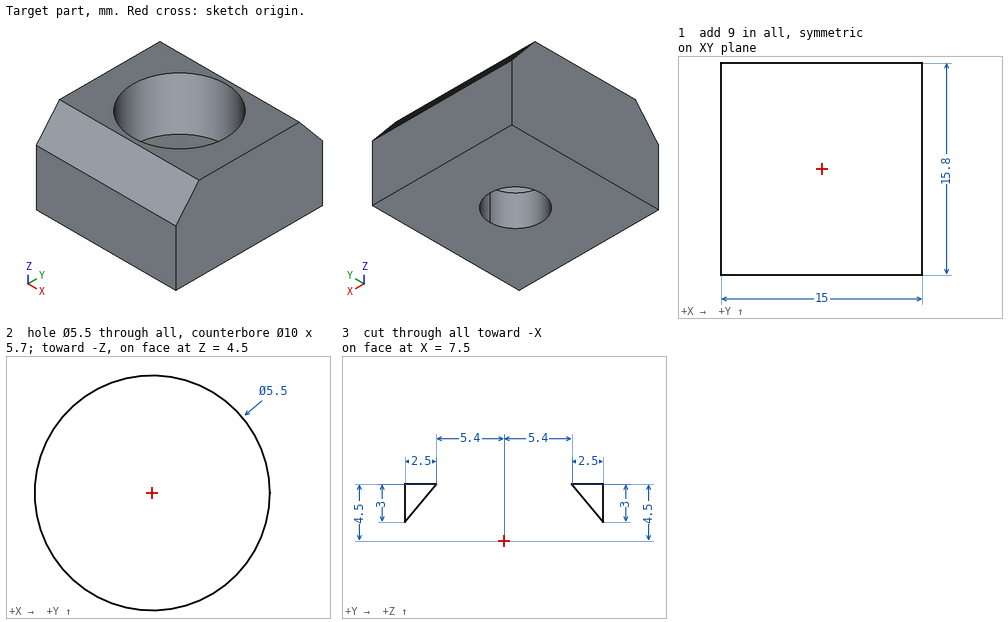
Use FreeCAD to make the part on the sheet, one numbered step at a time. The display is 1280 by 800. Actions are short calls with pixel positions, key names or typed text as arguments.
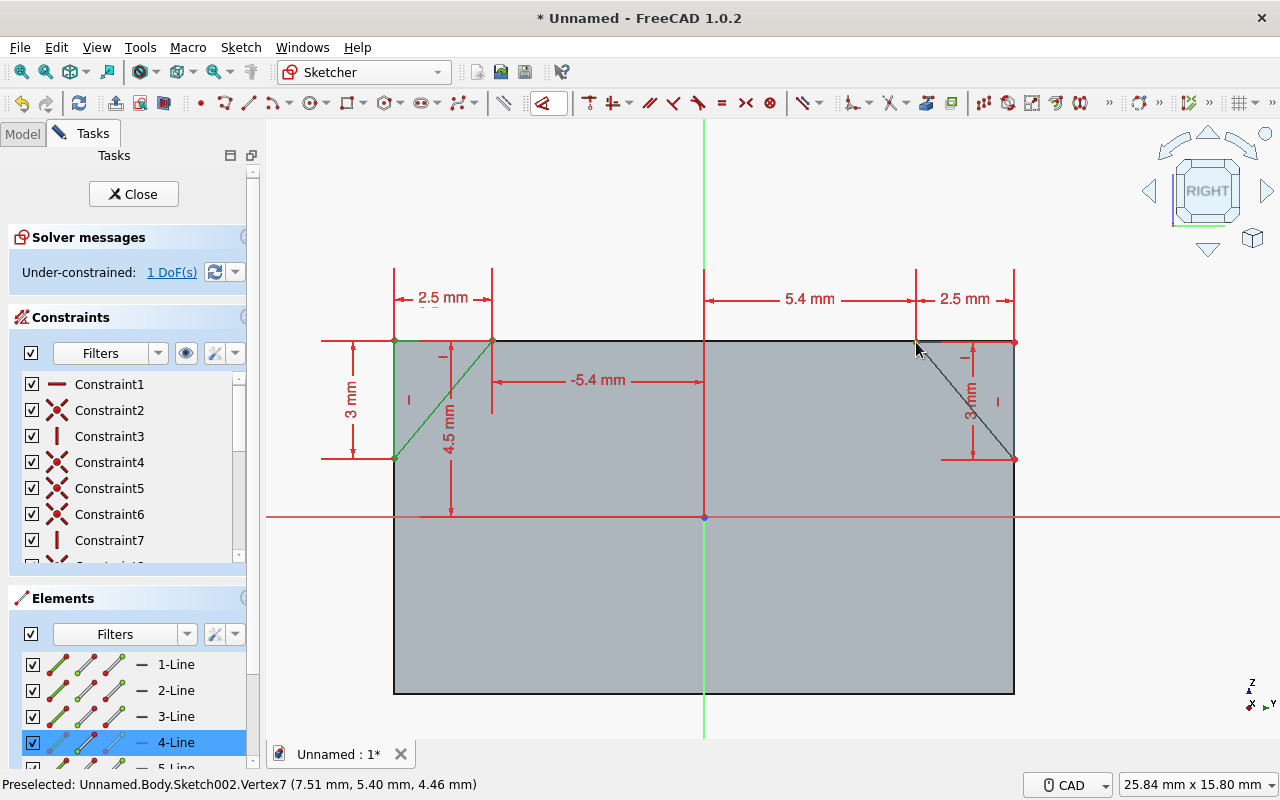
key(i)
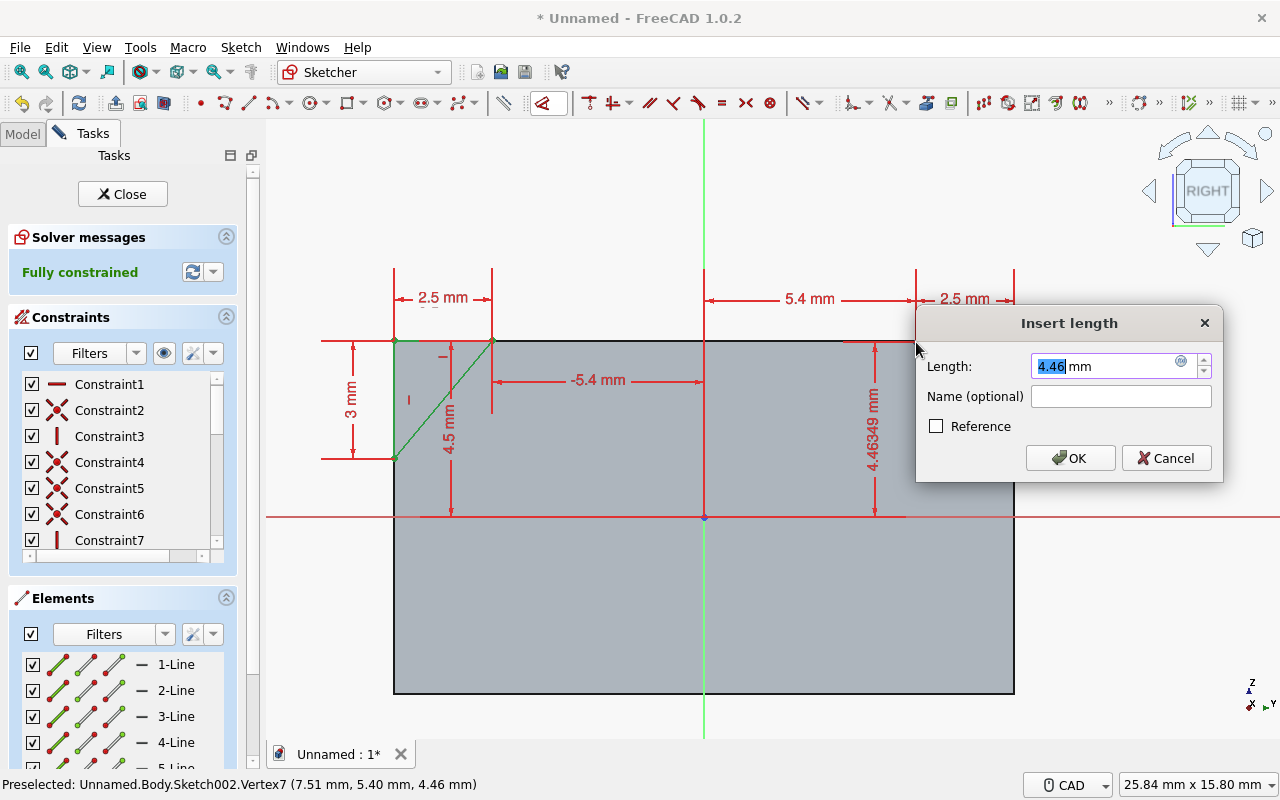
text(4.5)
key(Return)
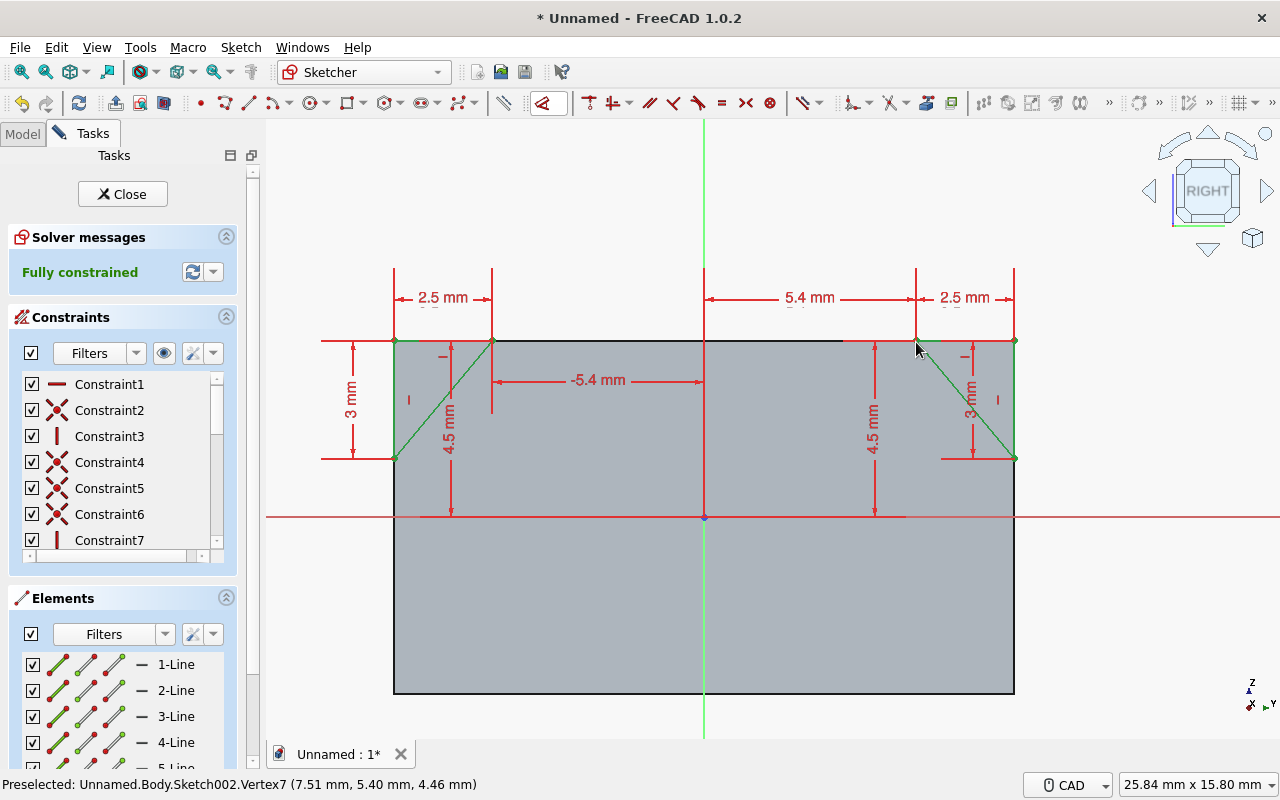
click(123, 194)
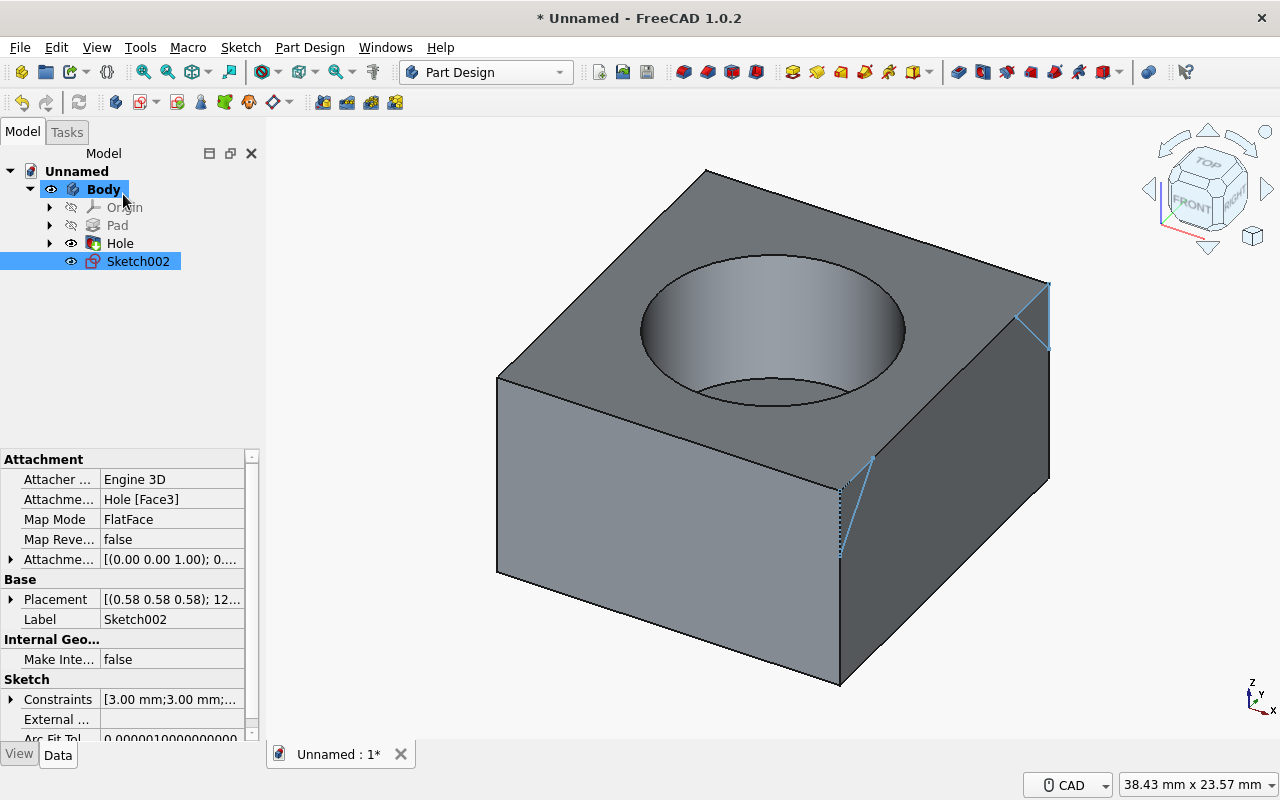
click(960, 72)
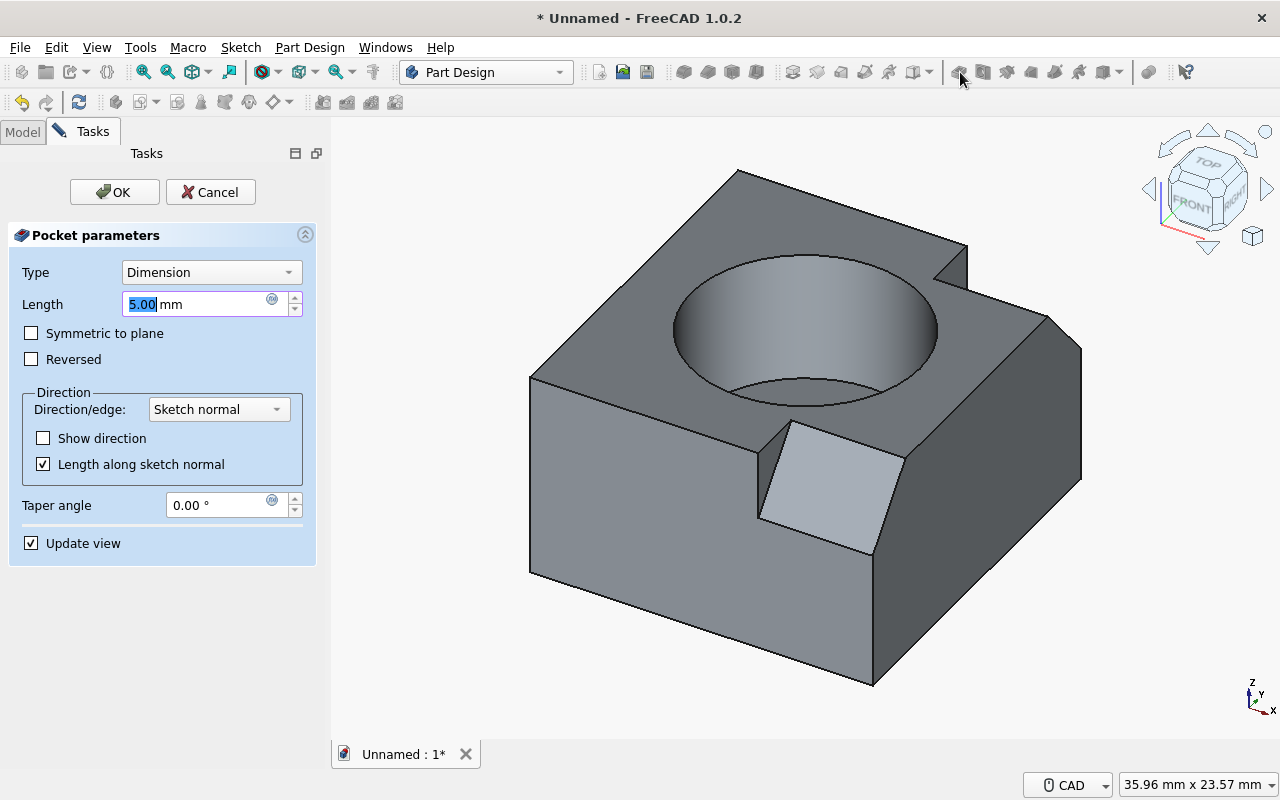
click(212, 272)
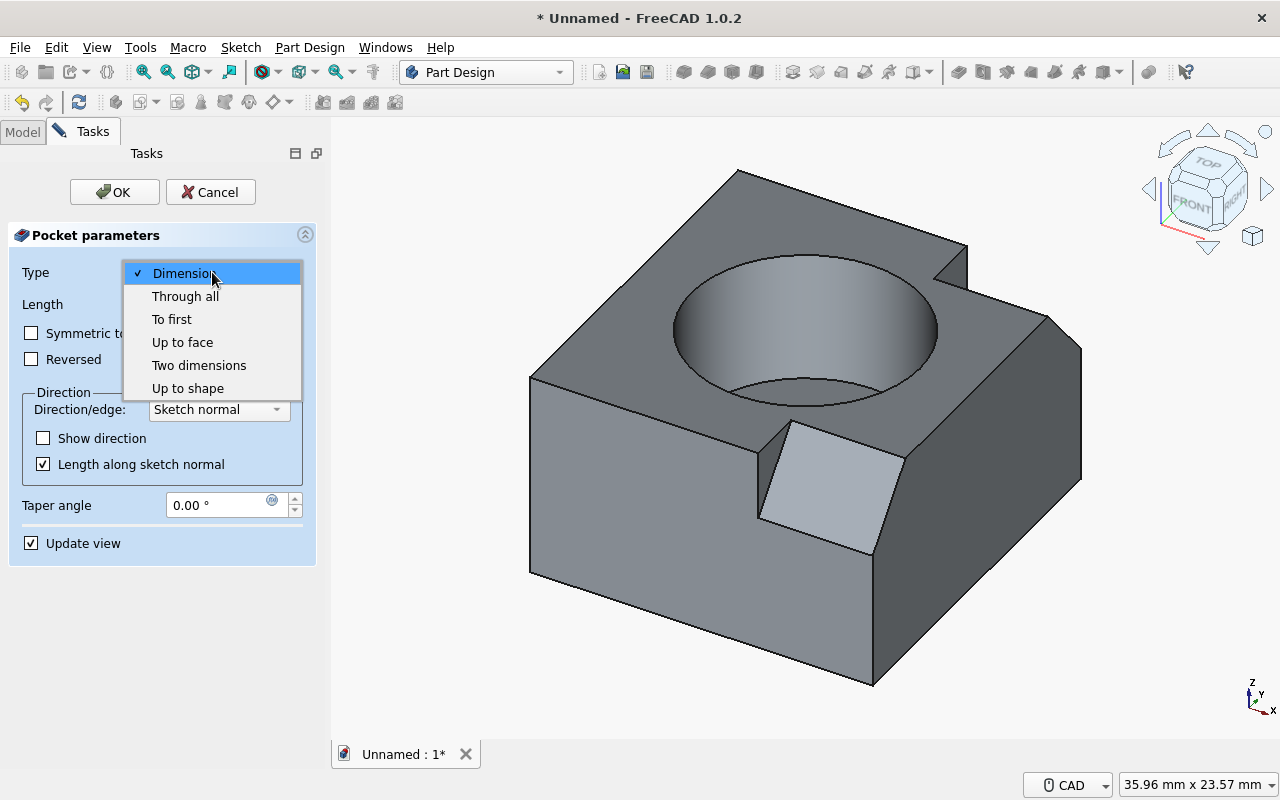
click(212, 296)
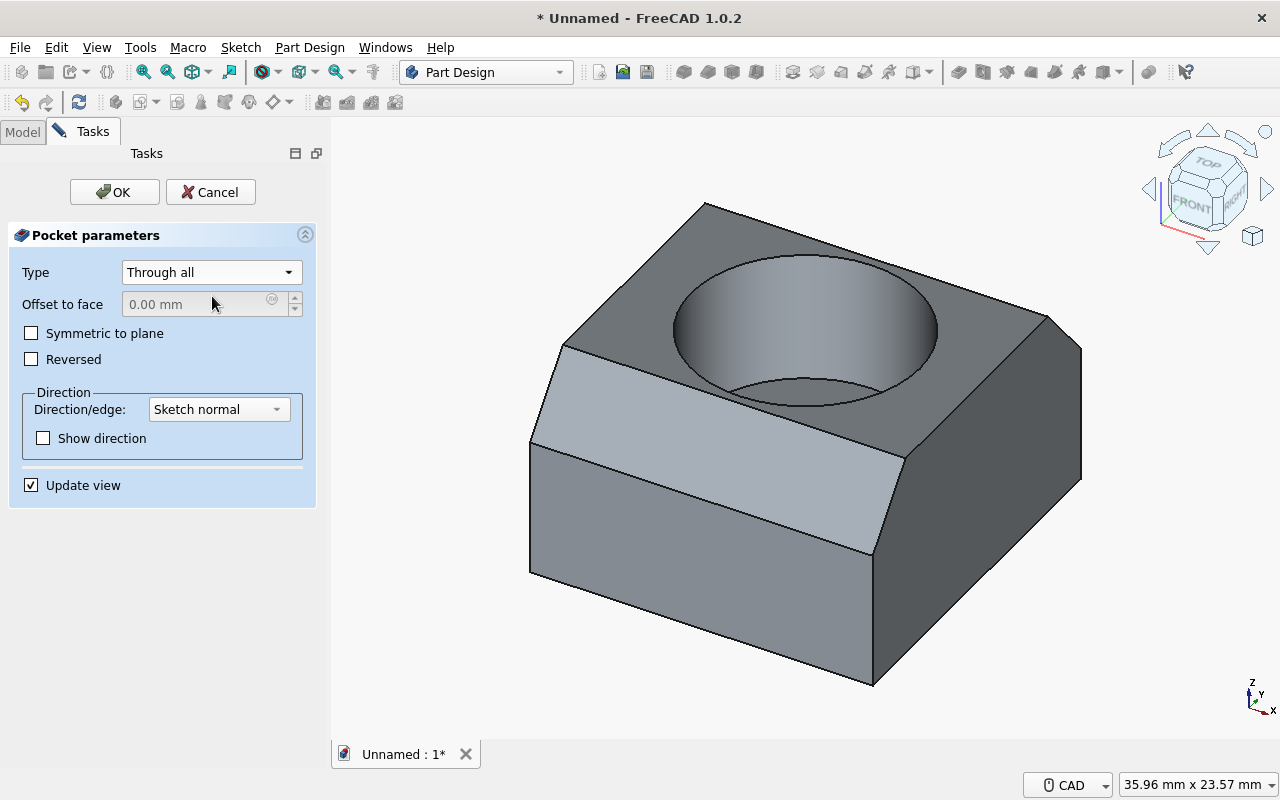
click(115, 192)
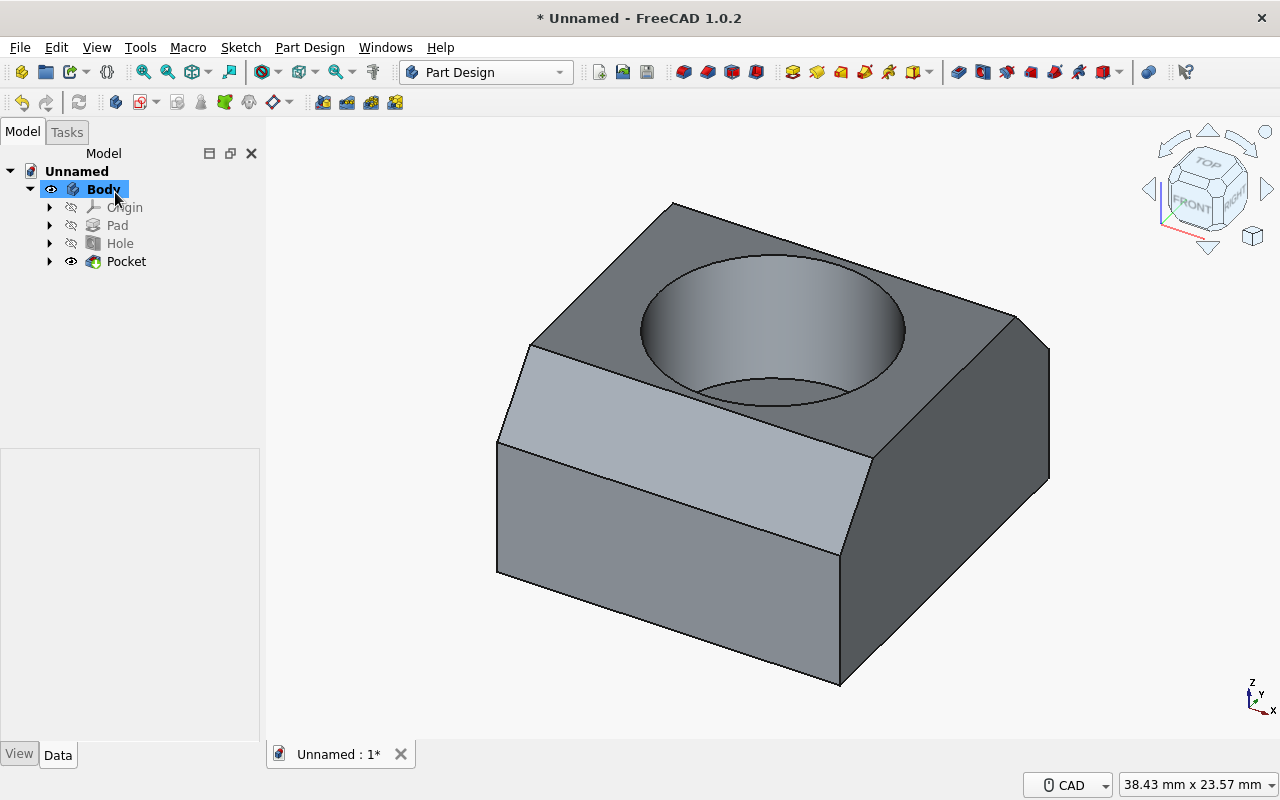
key(0)